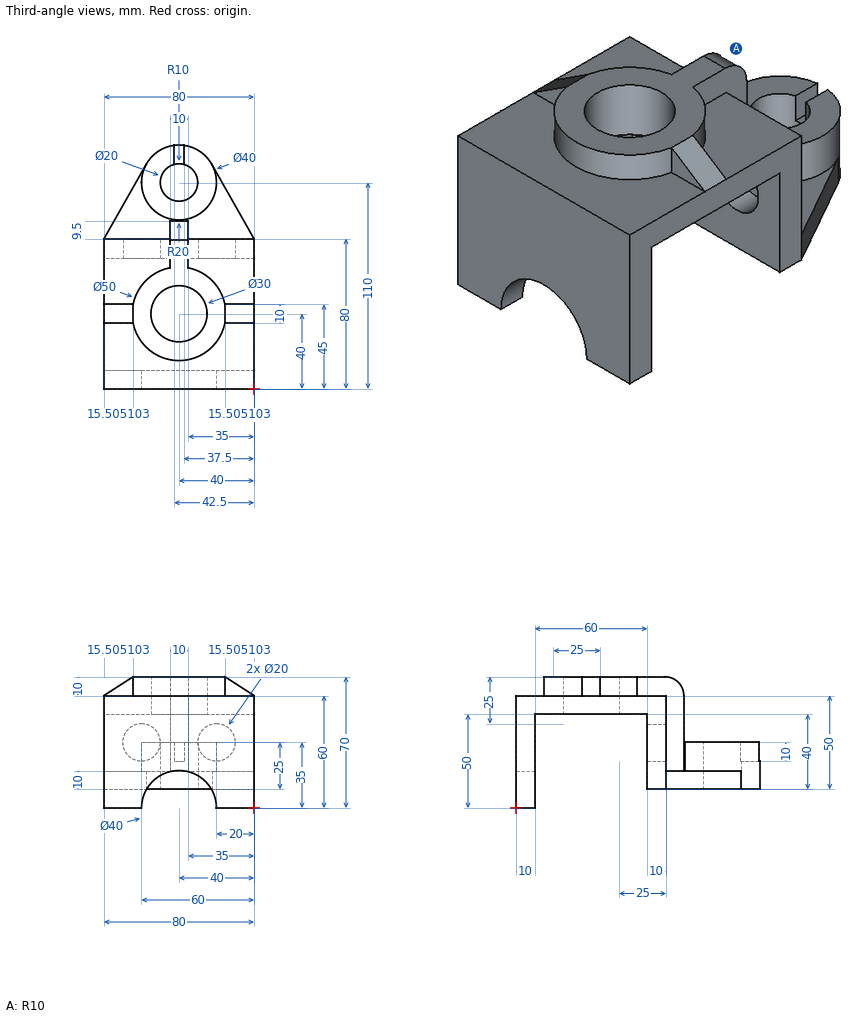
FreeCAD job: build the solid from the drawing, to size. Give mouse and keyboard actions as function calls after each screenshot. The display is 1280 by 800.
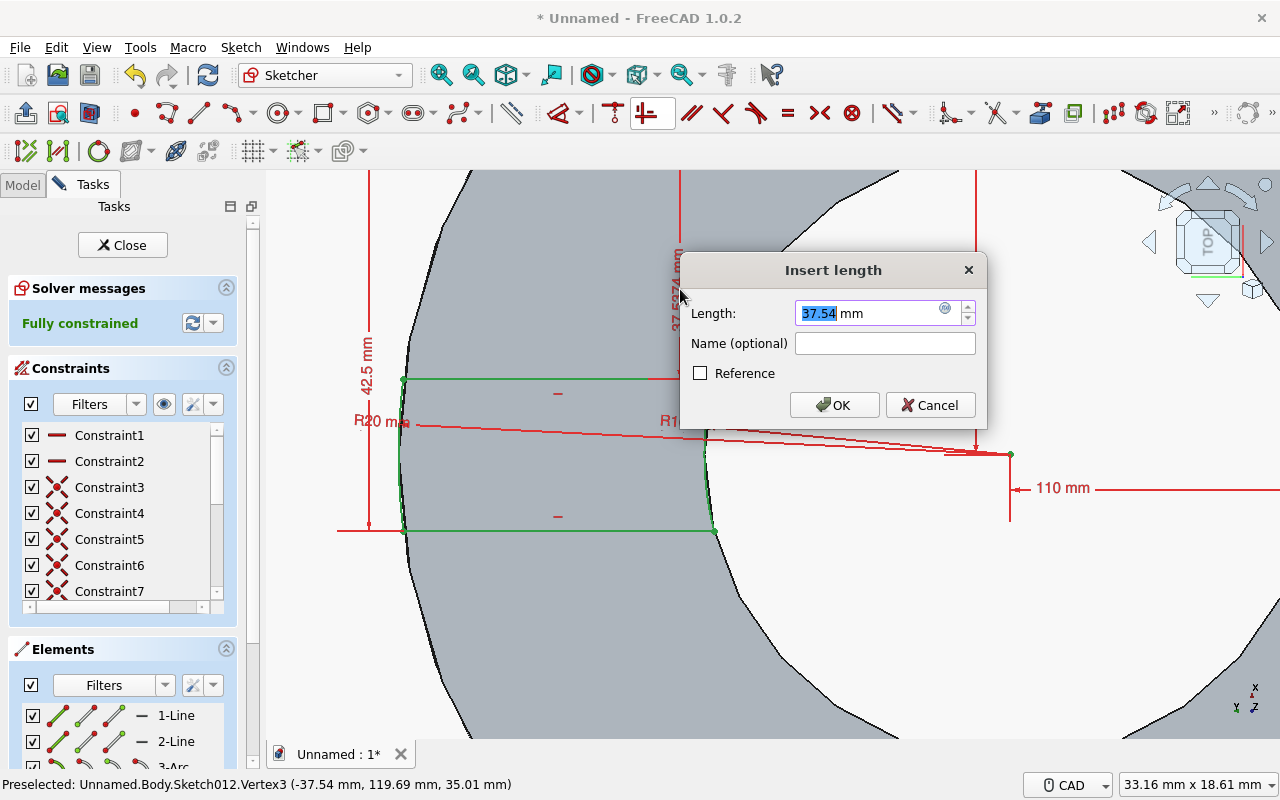
text(37.5)
key(Return)
key(Escape)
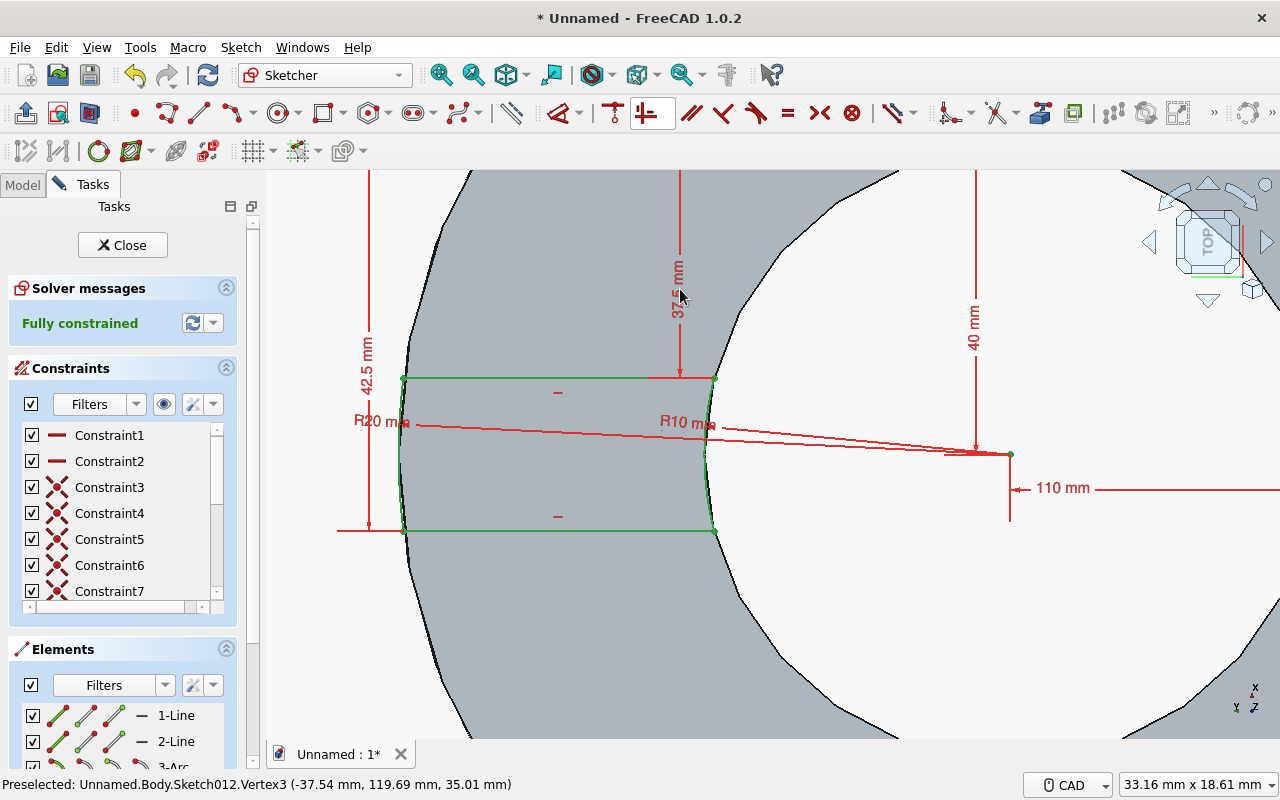
click(123, 245)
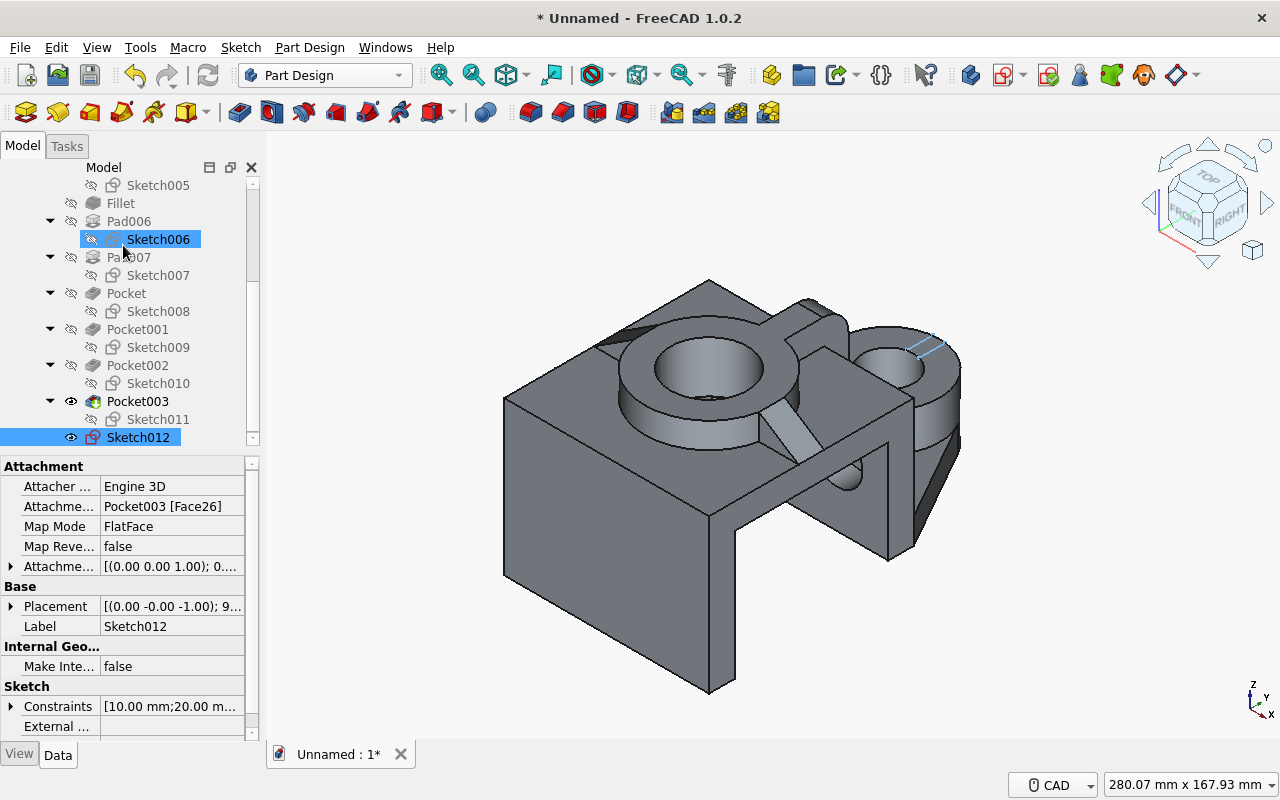
click(240, 112)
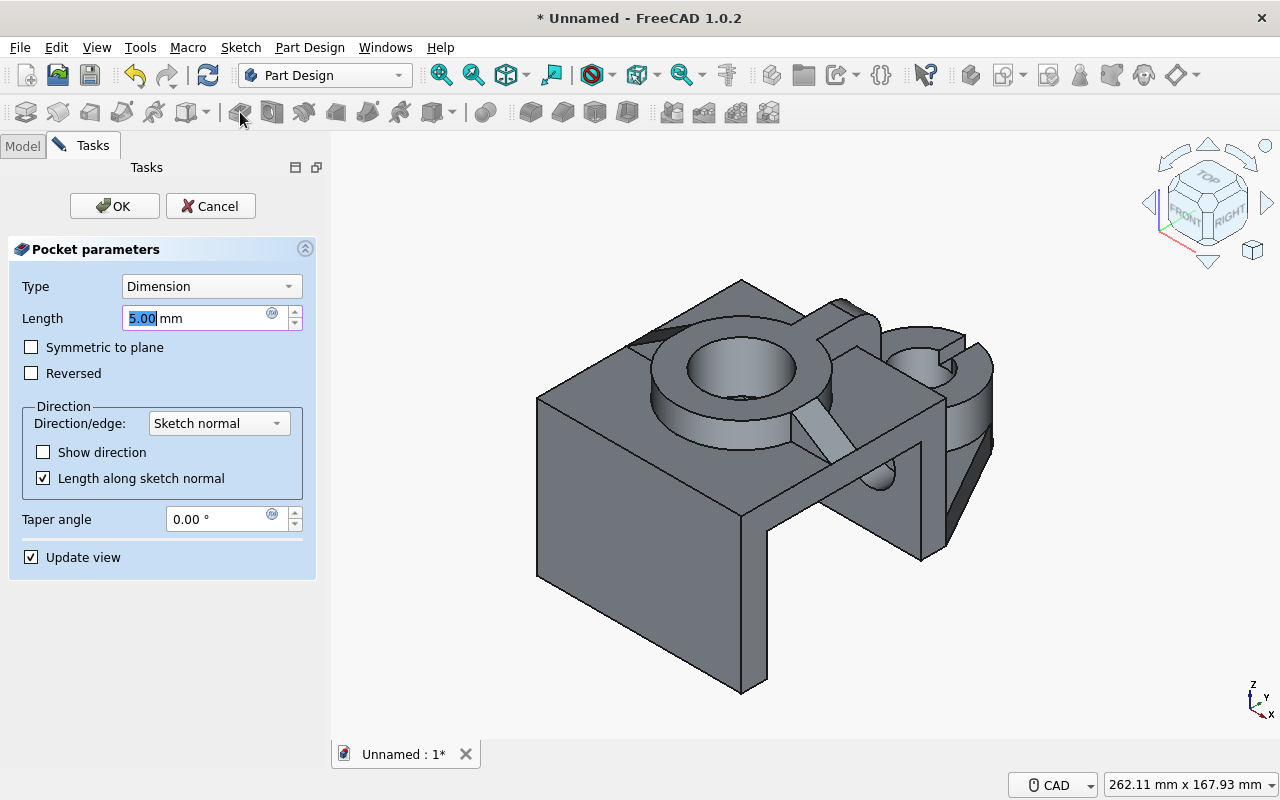
text(10)
key(Tab)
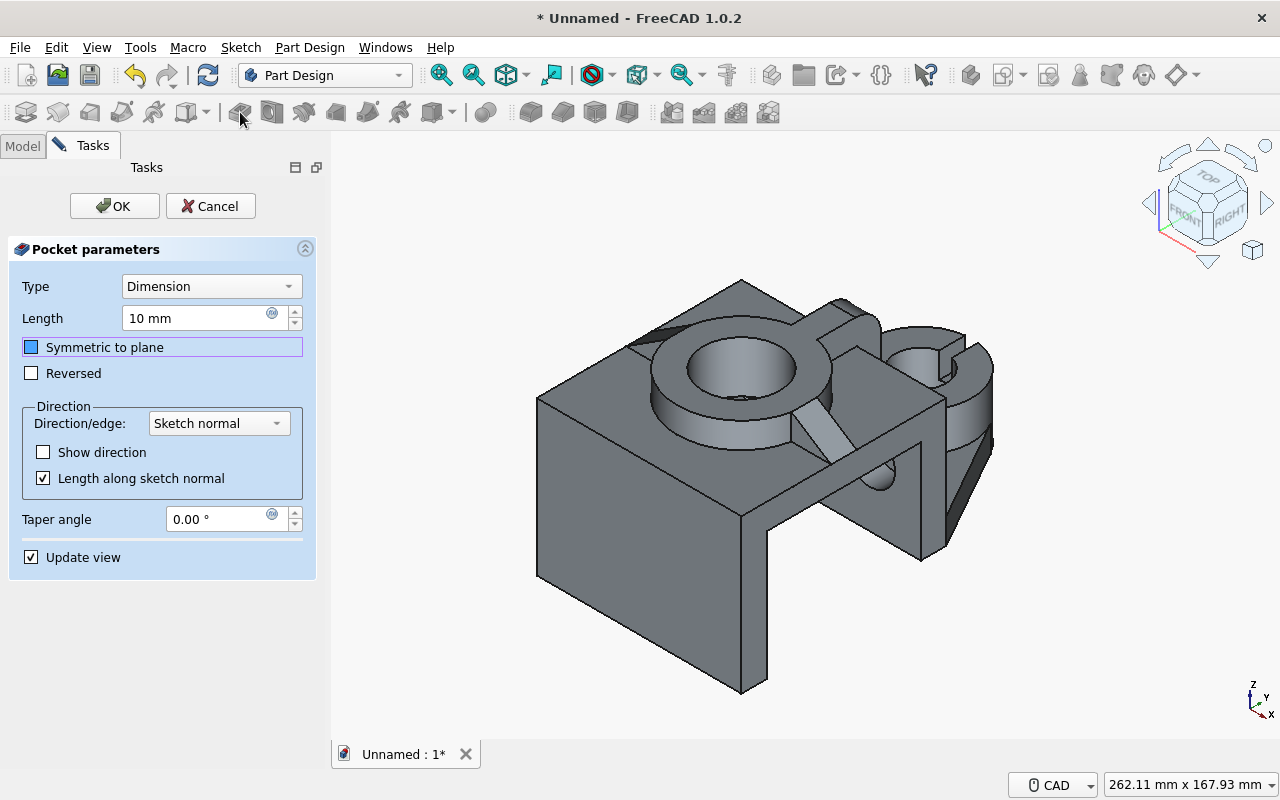
click(115, 206)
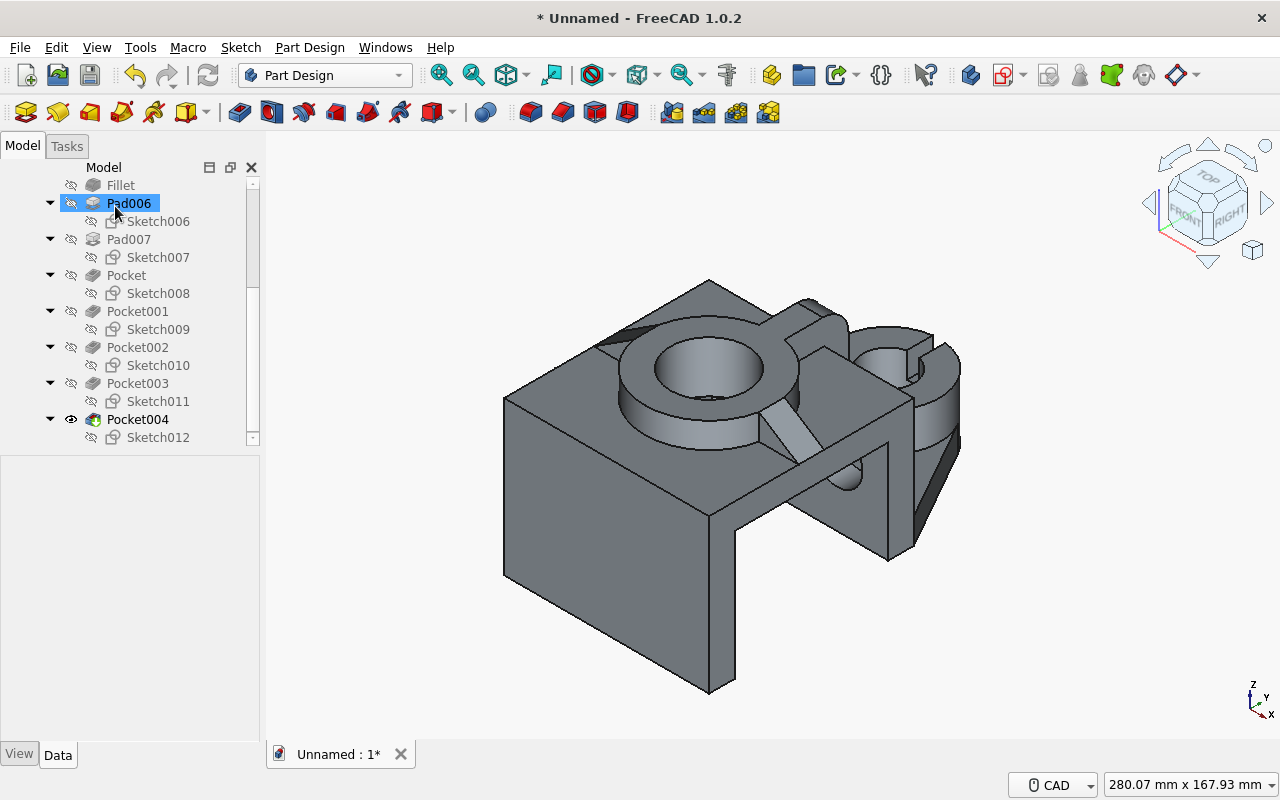
scroll(140, 307, down, 3)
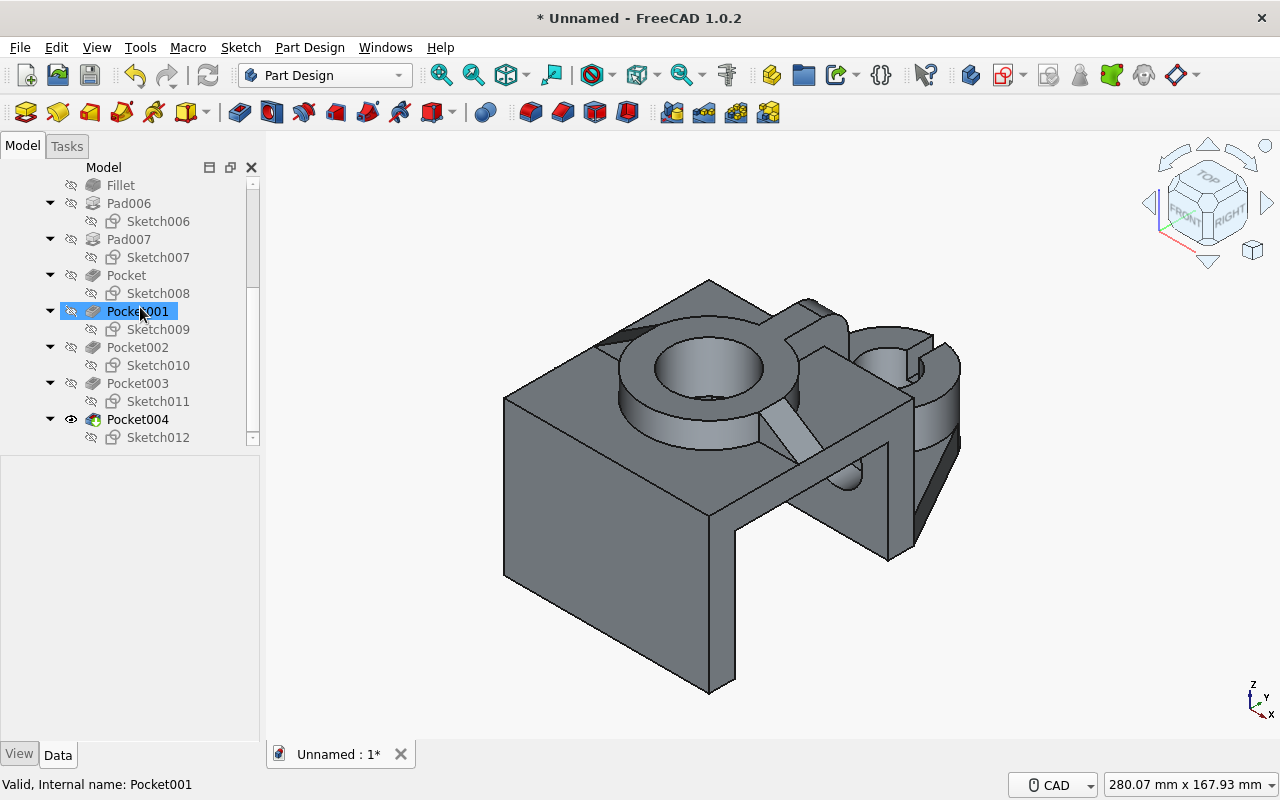
scroll(140, 307, up, 15)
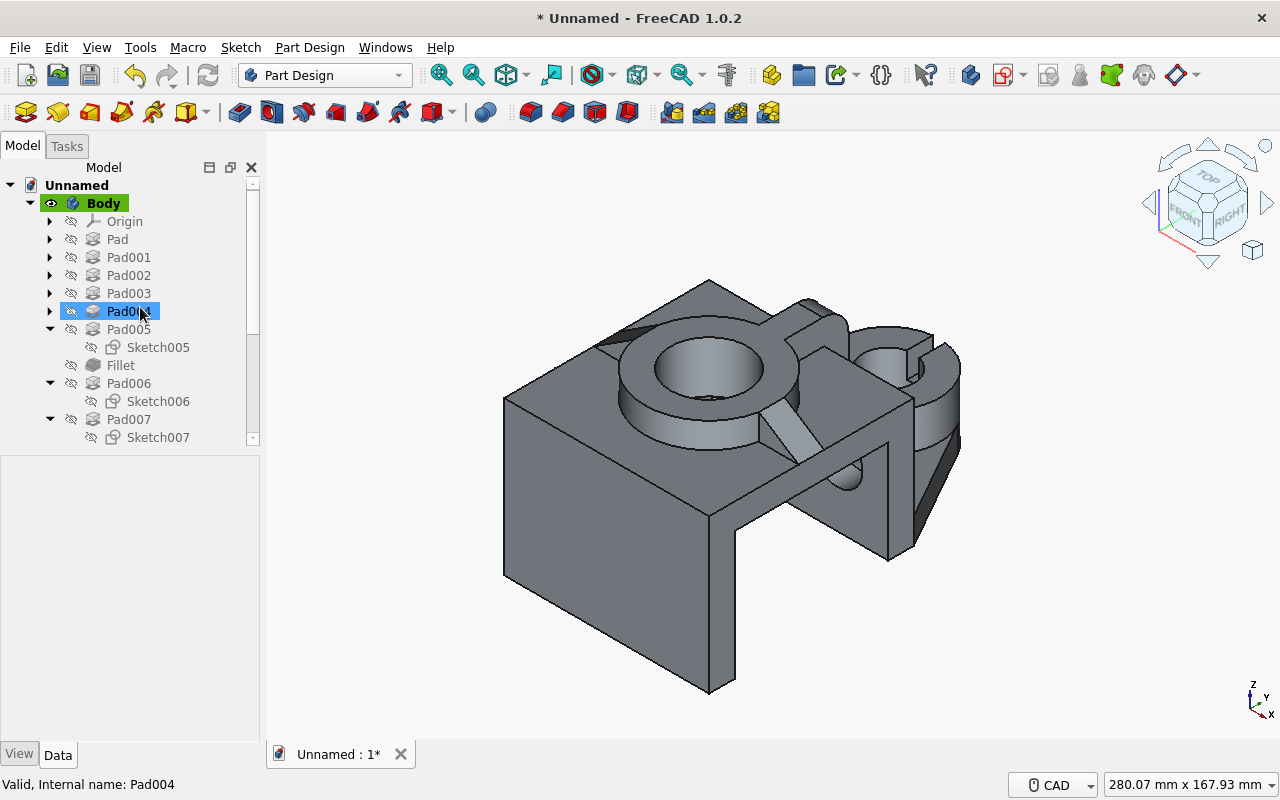
click(50, 221)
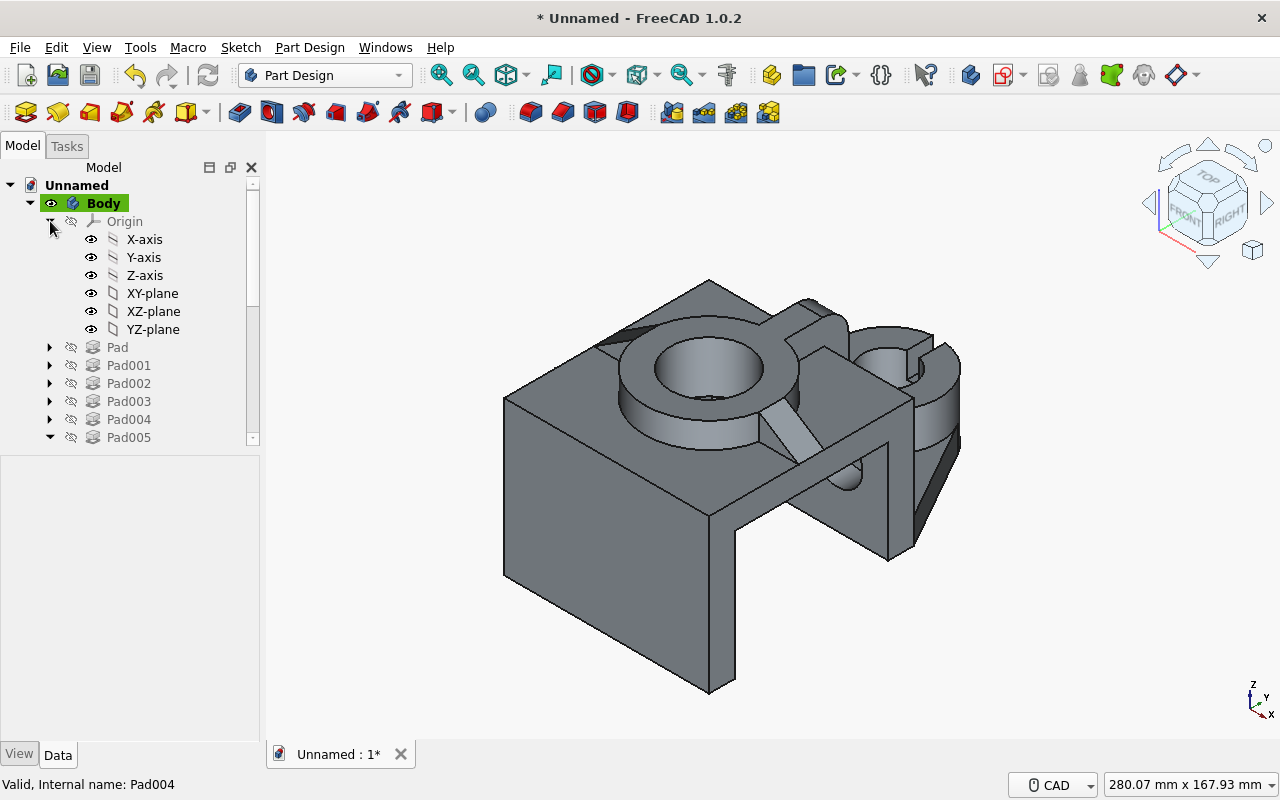
click(136, 311)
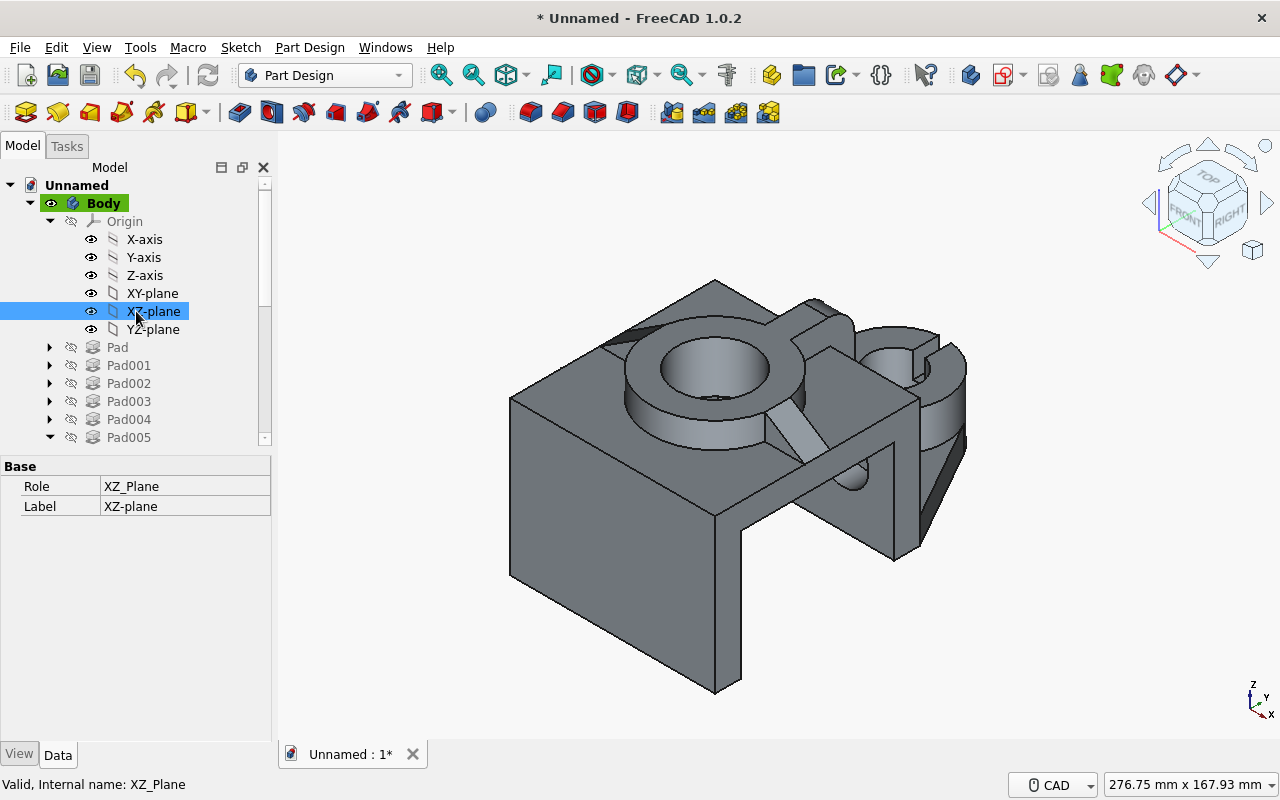
click(1176, 76)